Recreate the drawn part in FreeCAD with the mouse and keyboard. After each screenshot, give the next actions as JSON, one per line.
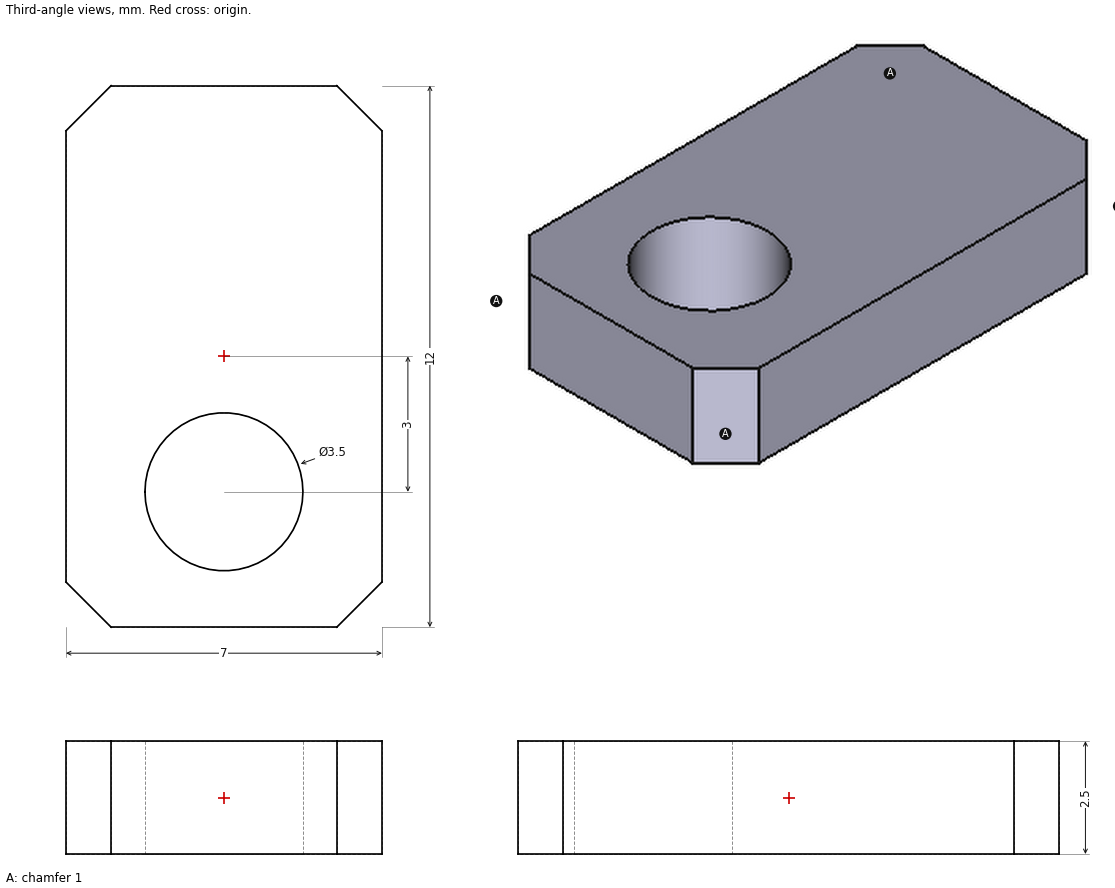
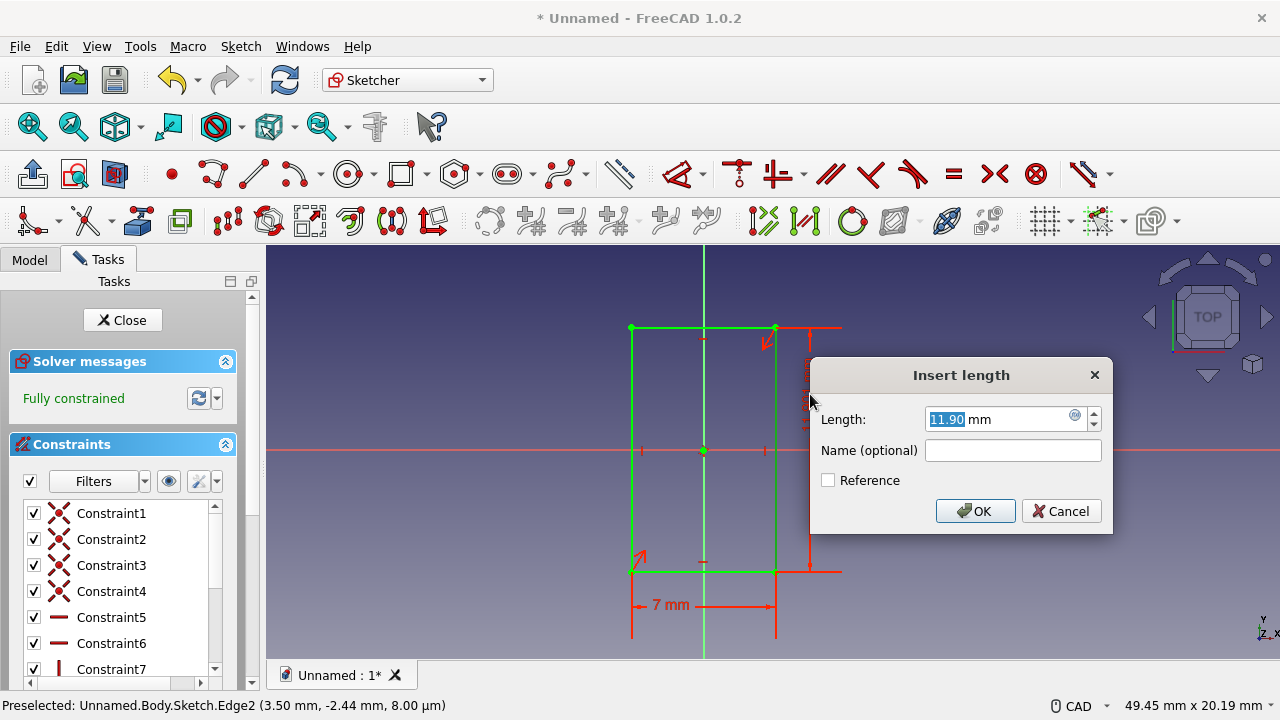
{"action": "type", "text": "12"}
{"action": "key", "text": "Return"}
{"action": "key", "text": "Escape"}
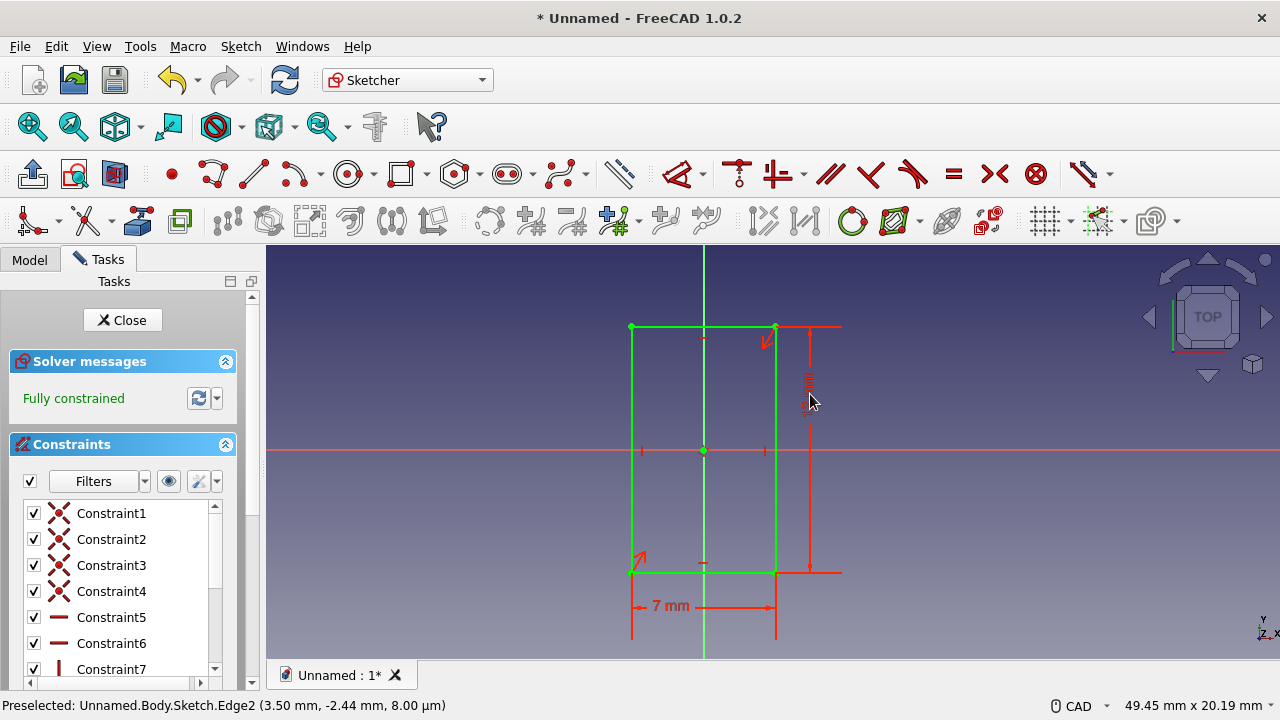
{"action": "left_click", "coordinate": [123, 320]}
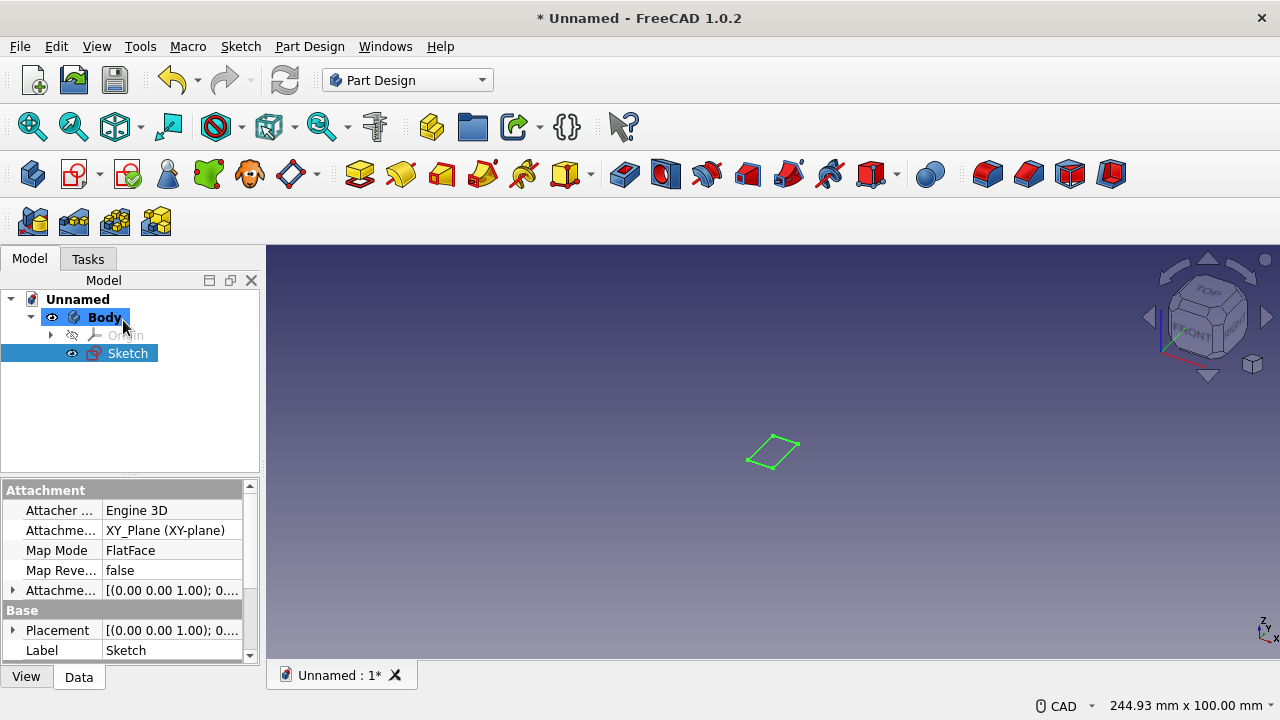
{"action": "left_click", "coordinate": [360, 174]}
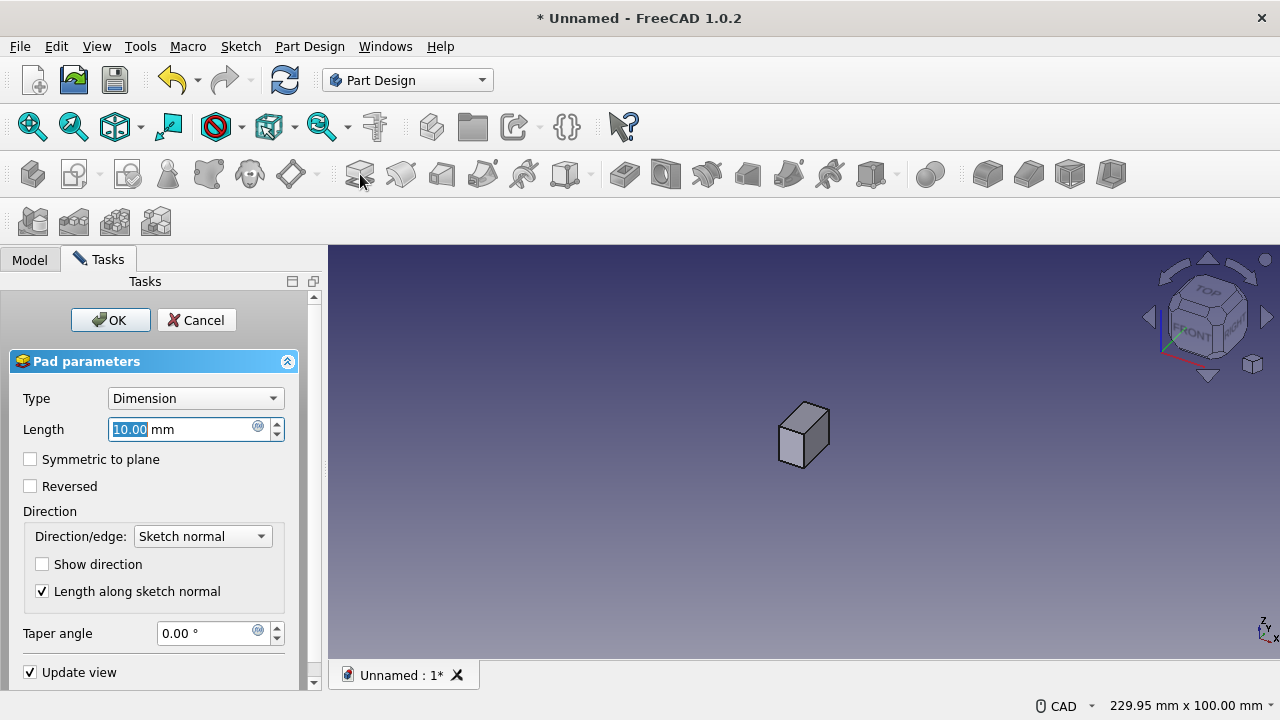
{"action": "type", "text": "2.5"}
{"action": "key", "text": "Tab"}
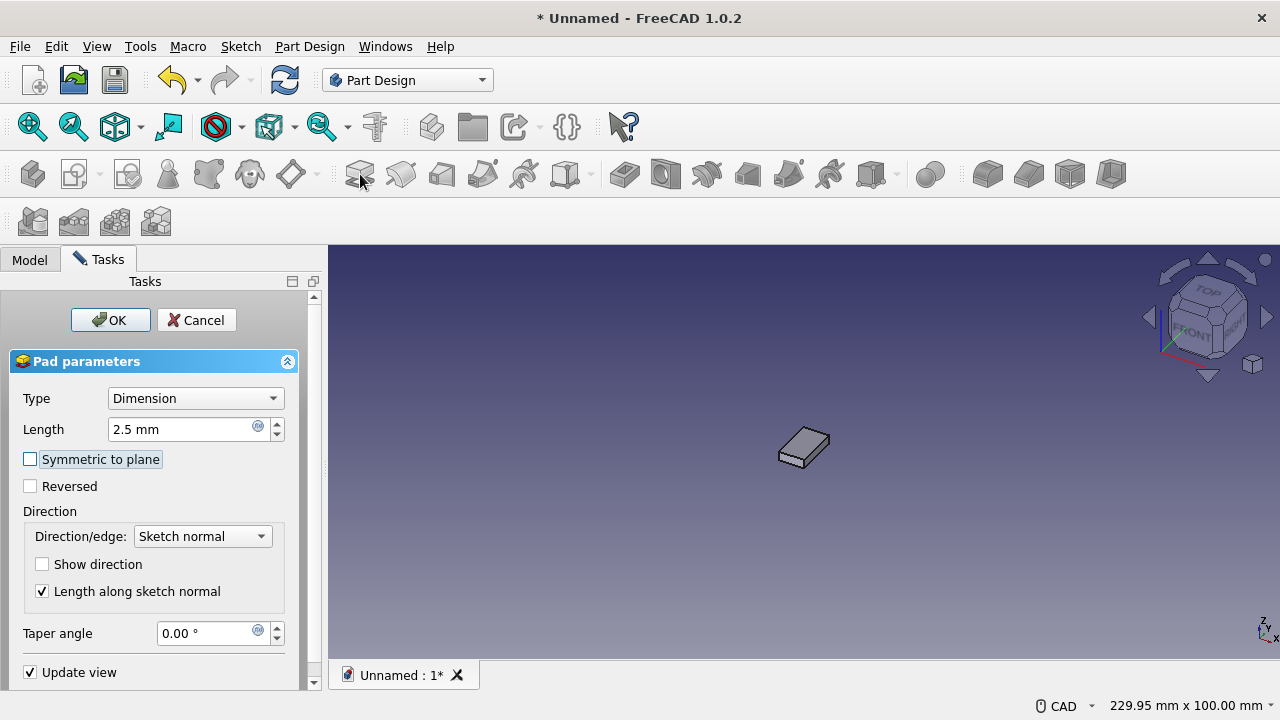
{"action": "left_click", "coordinate": [31, 459]}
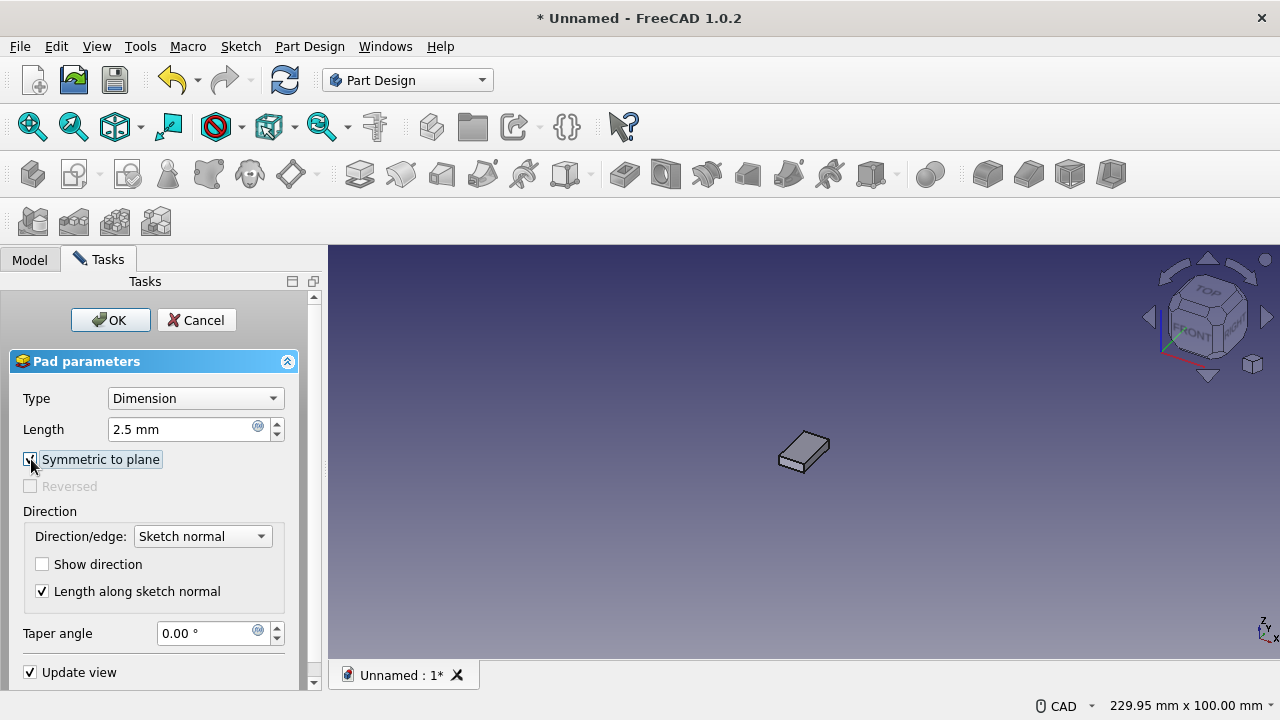
{"action": "left_click", "coordinate": [111, 320]}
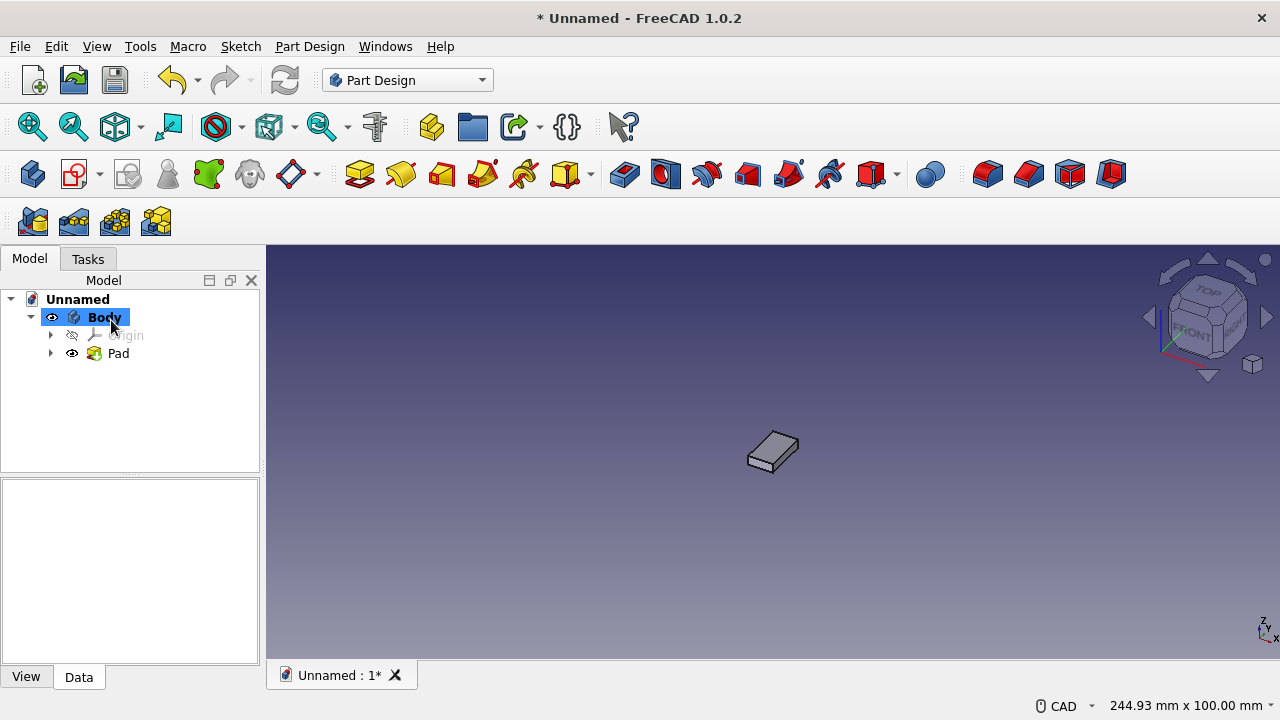
{"action": "left_click", "coordinate": [33, 128]}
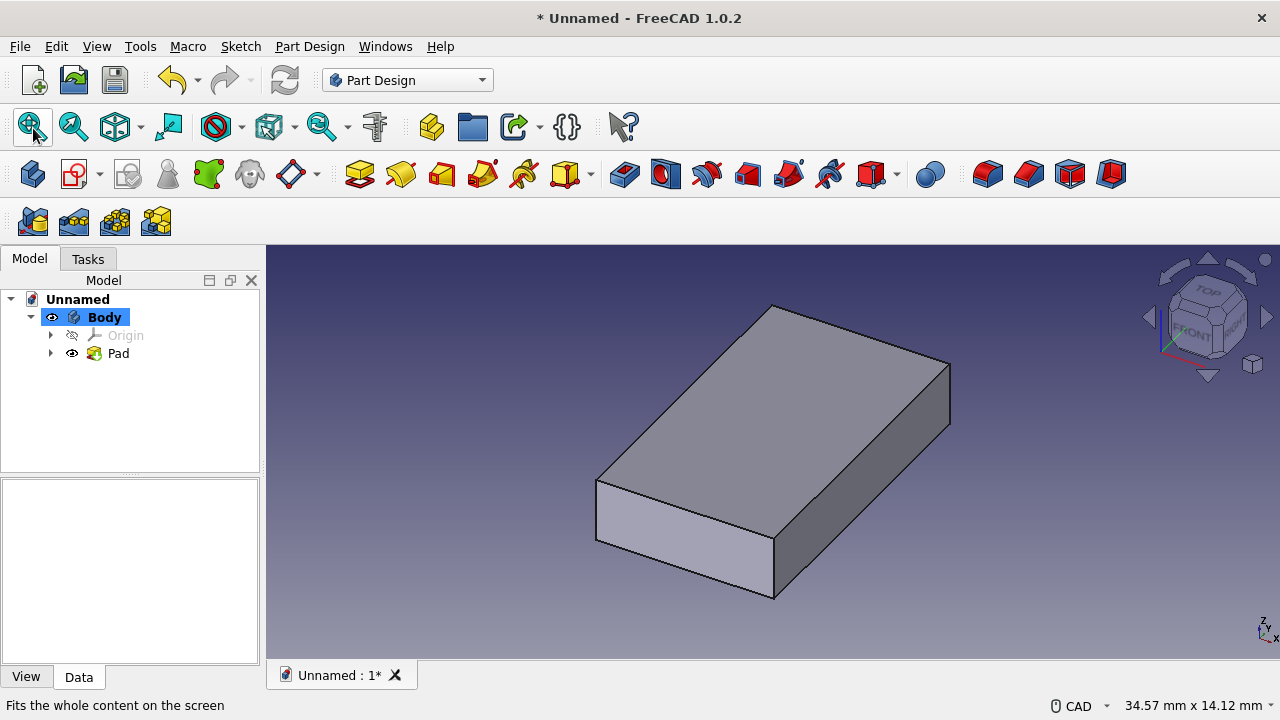
{"action": "left_click", "coordinate": [798, 396]}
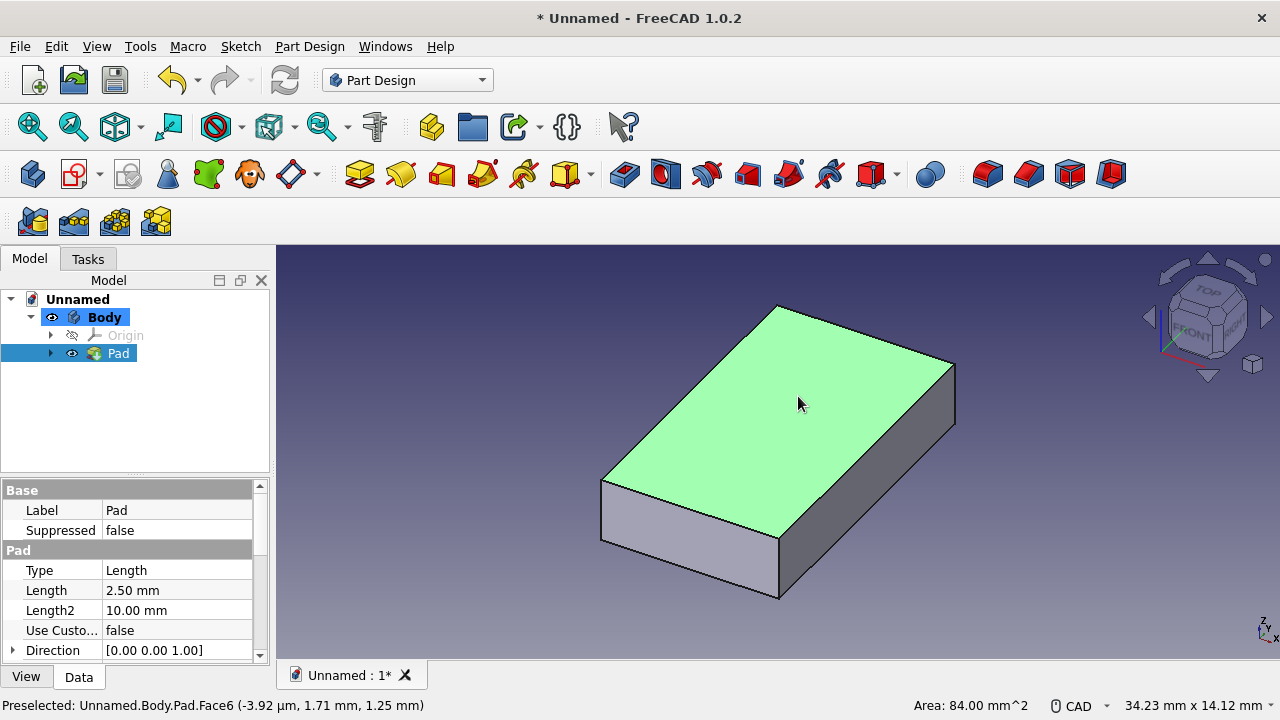
{"action": "left_click", "coordinate": [74, 174]}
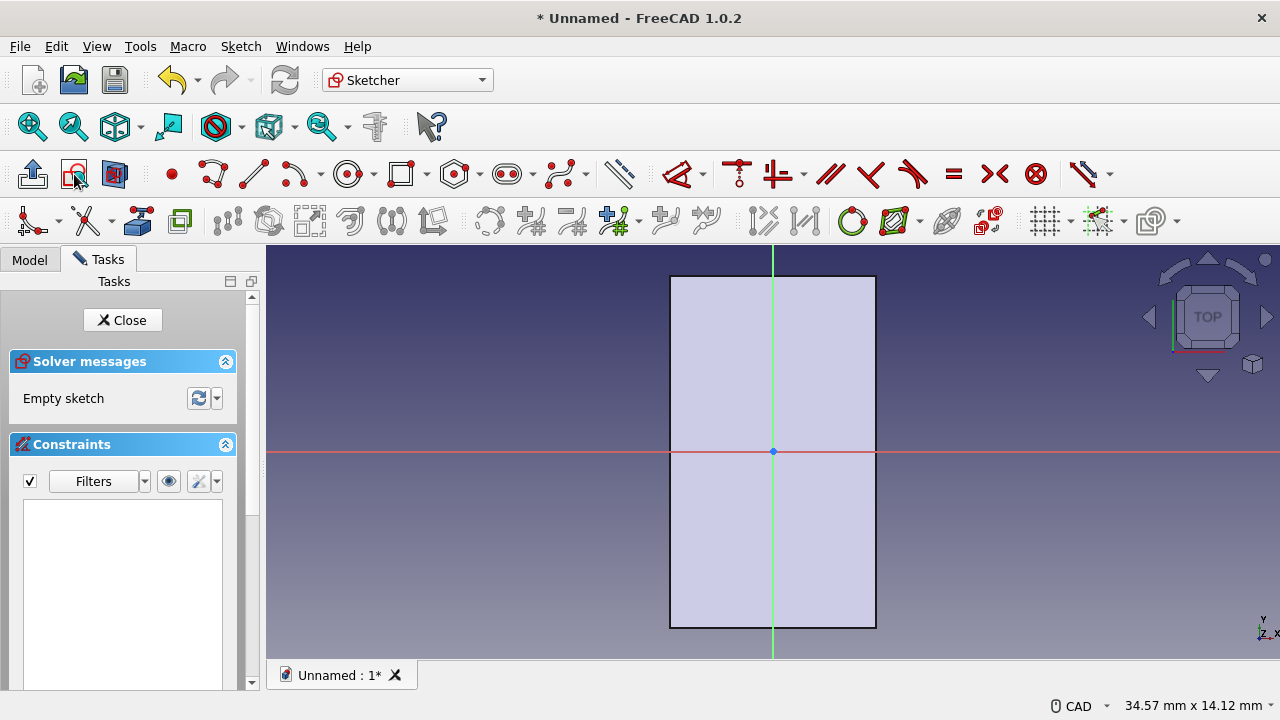
{"action": "scroll", "coordinate": [856, 606], "scroll_direction": "up", "scroll_amount": 3}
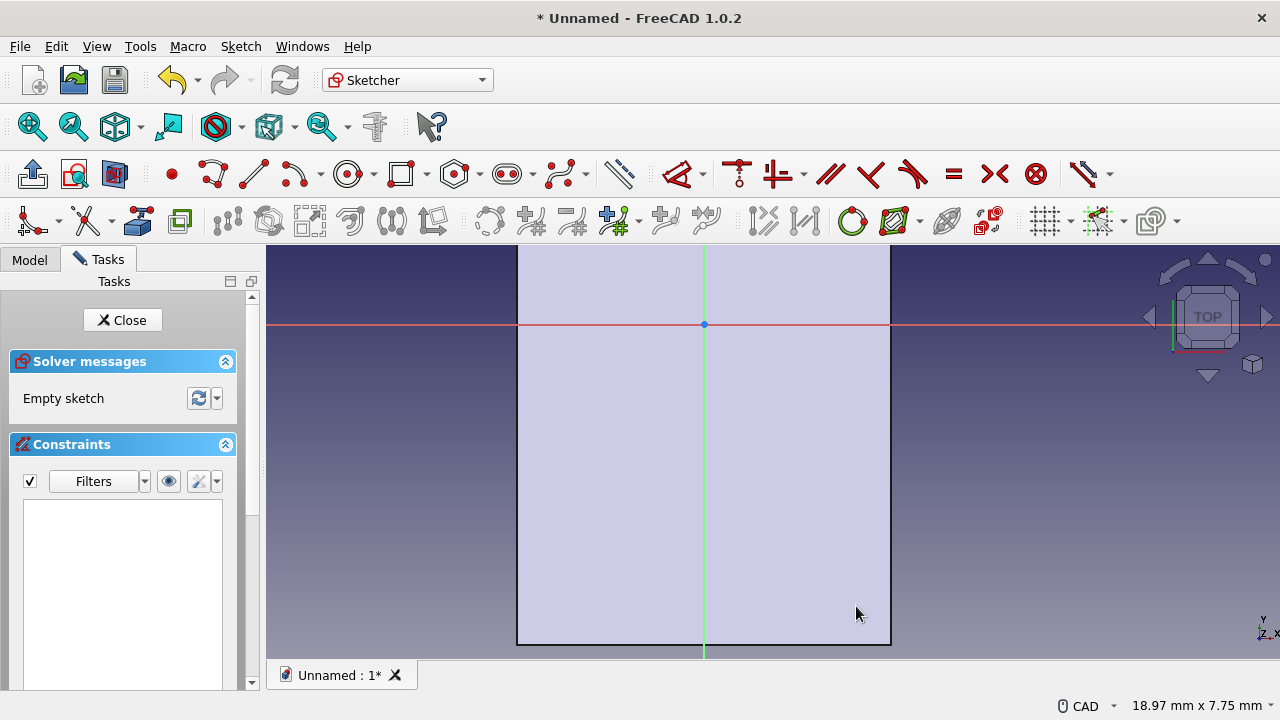
{"action": "key", "text": "g c"}